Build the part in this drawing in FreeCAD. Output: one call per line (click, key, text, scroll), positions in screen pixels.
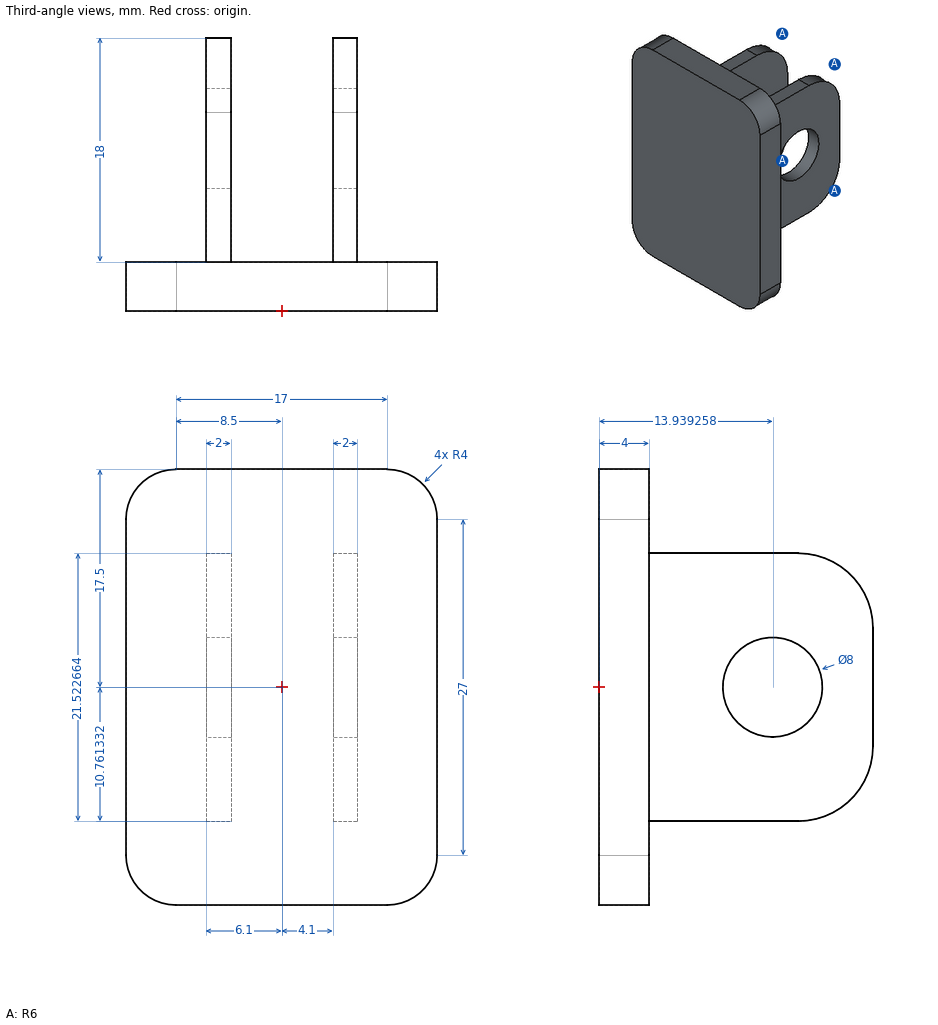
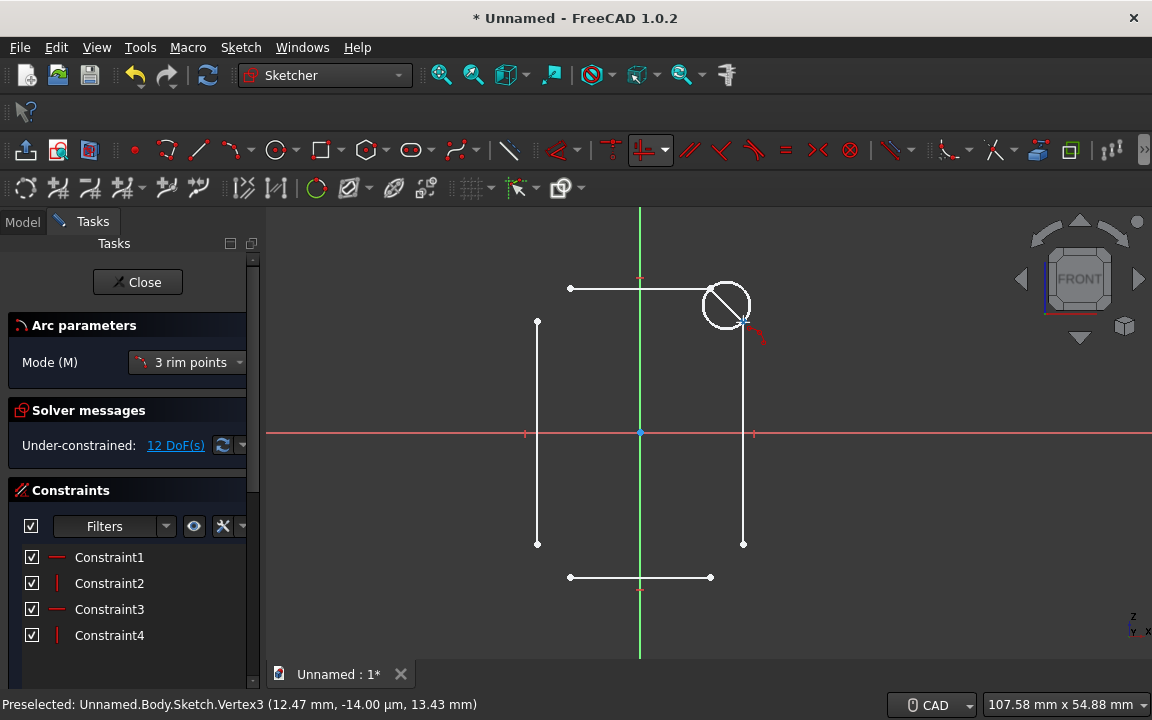
scroll(734, 298, up, 3)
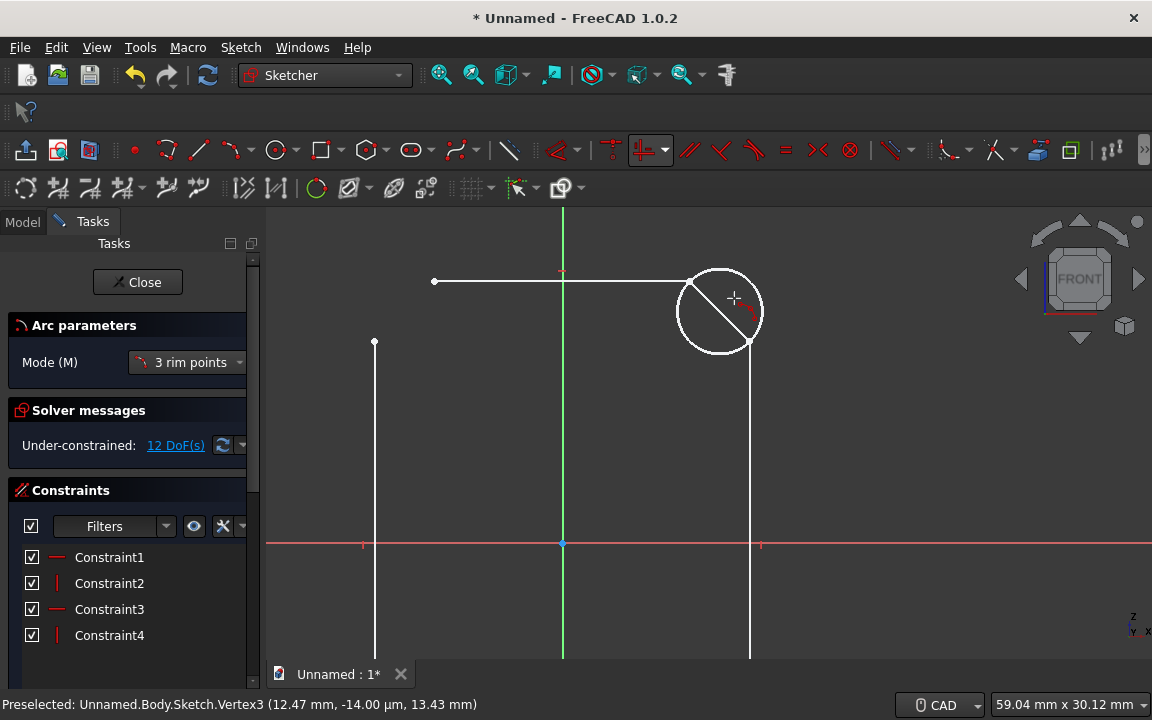
click(733, 298)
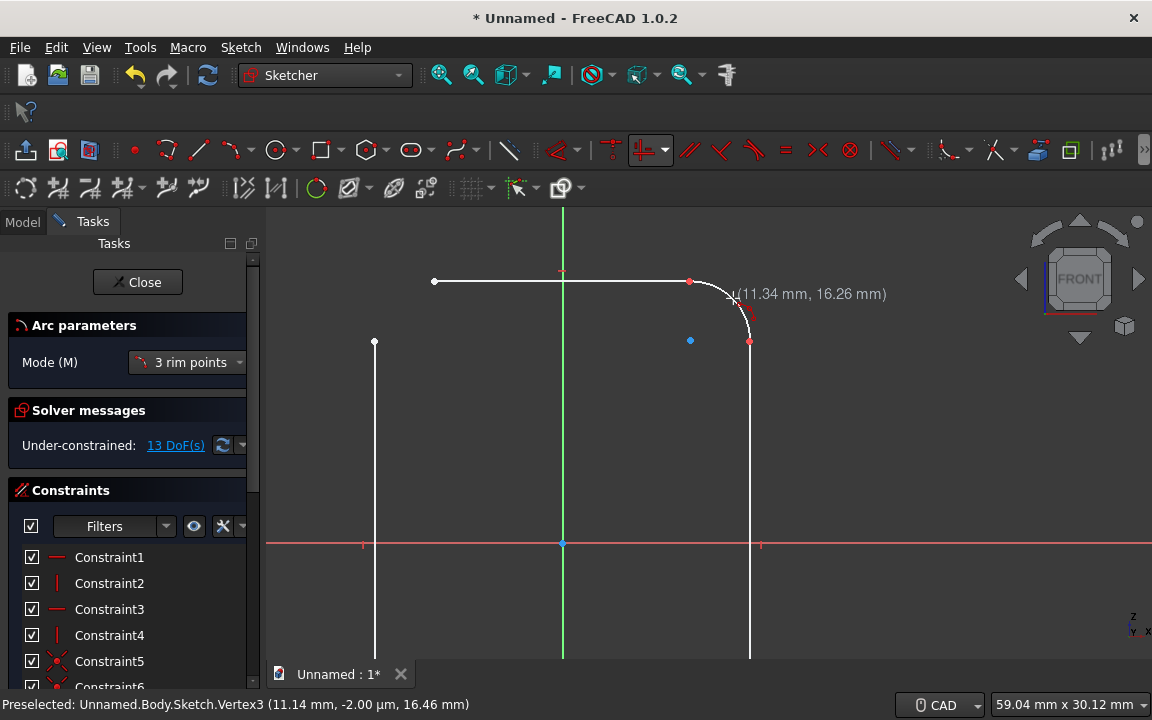
scroll(735, 299, down, 3)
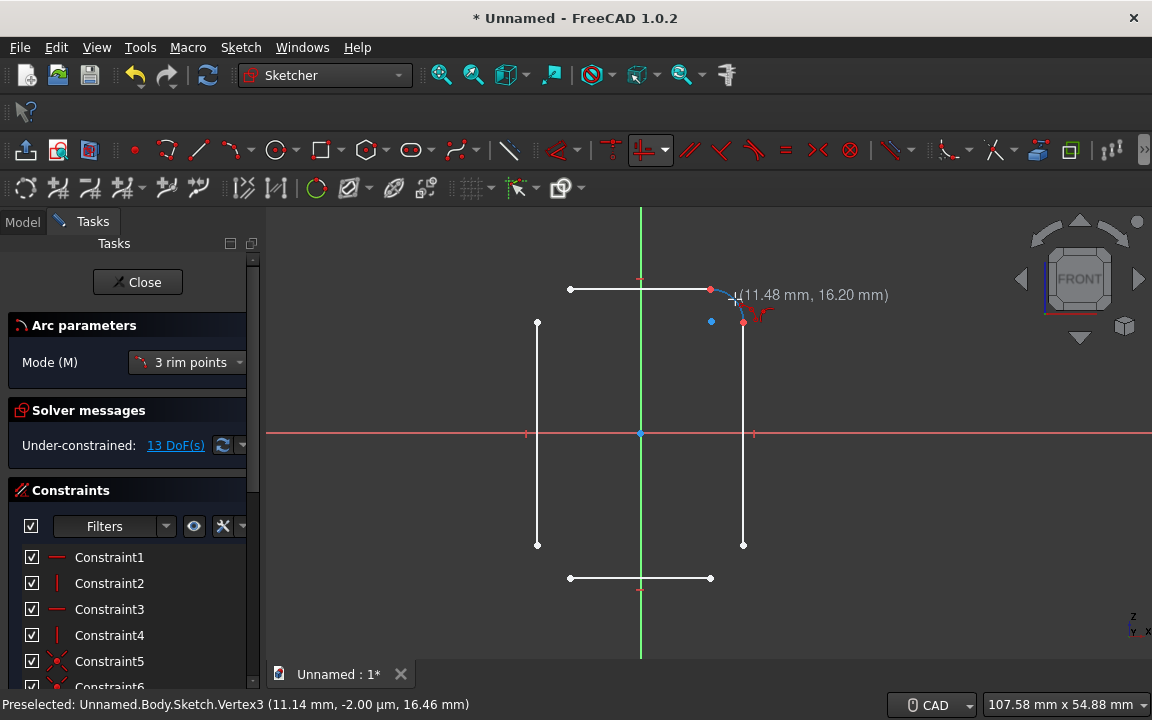
click(743, 545)
click(710, 578)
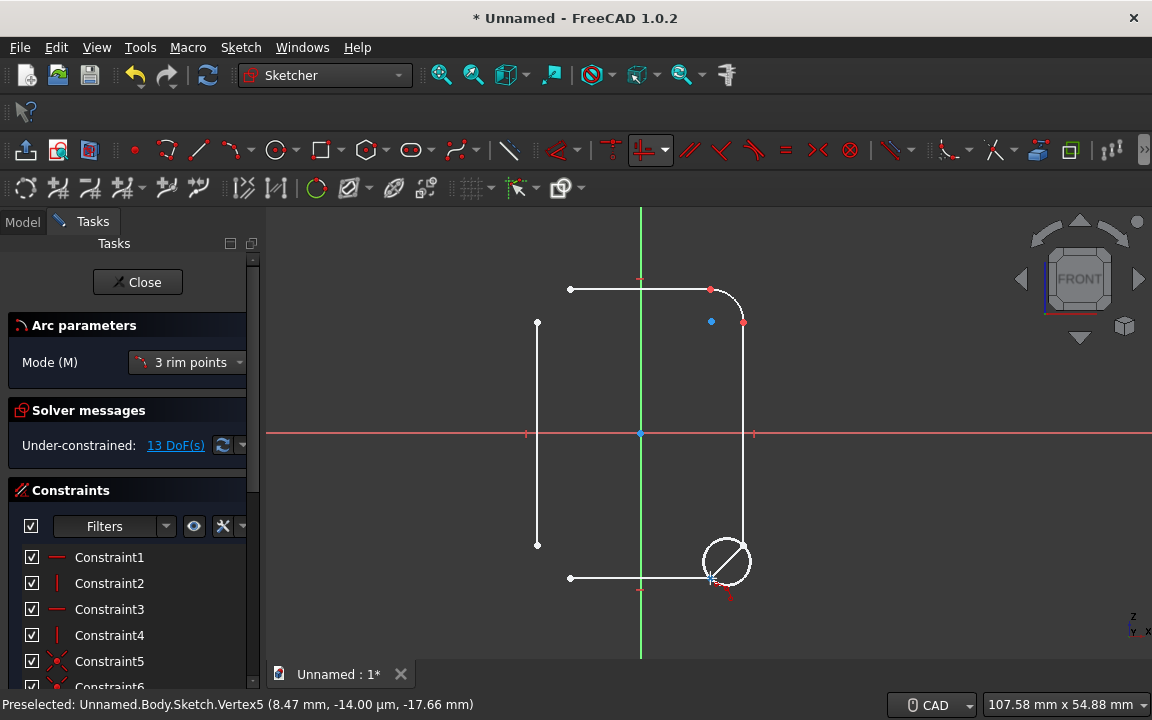
scroll(734, 568, up, 3)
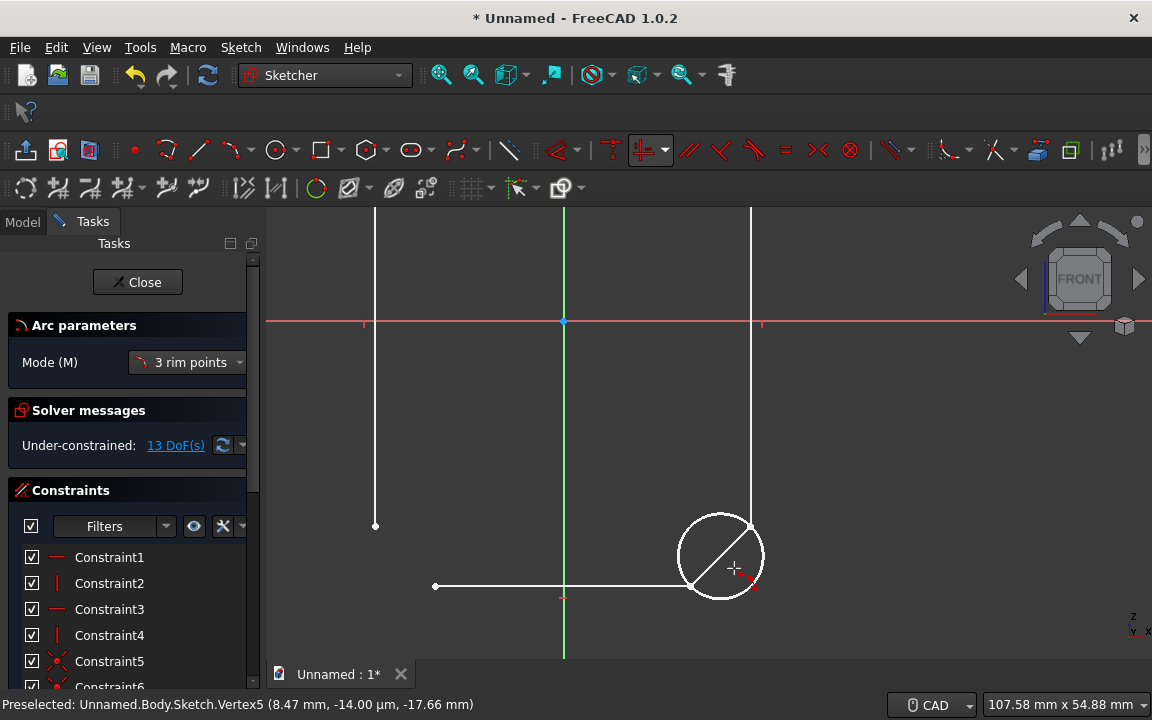
click(734, 566)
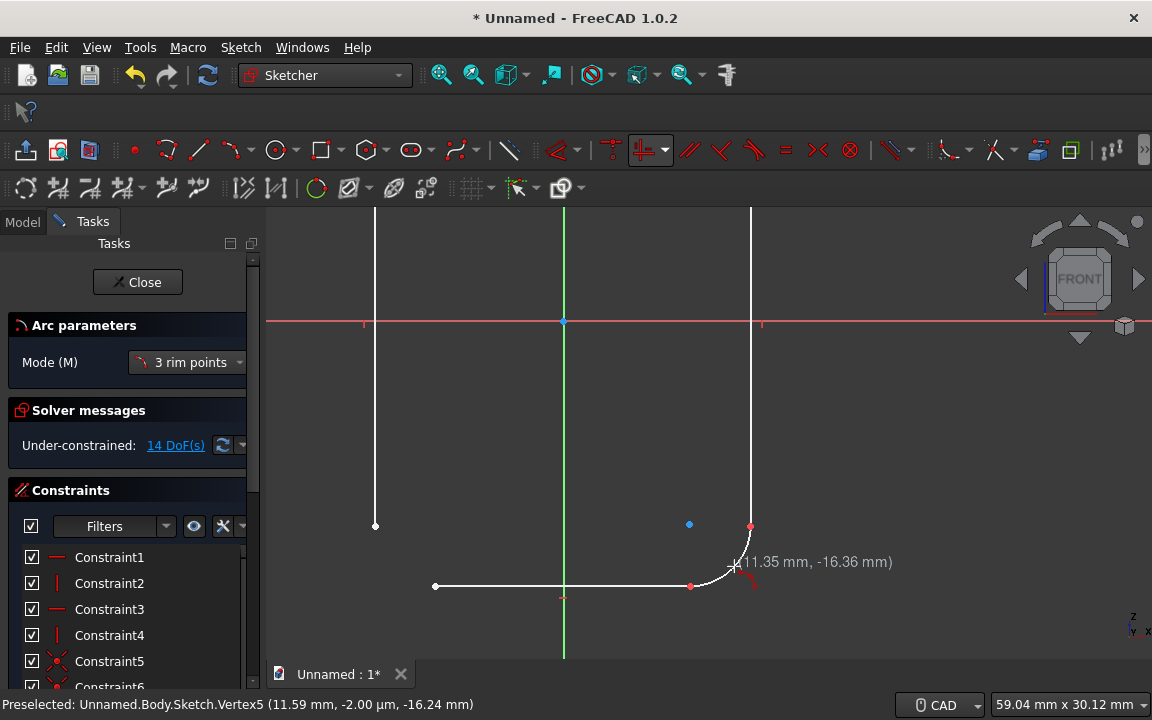
click(436, 586)
click(375, 526)
click(394, 566)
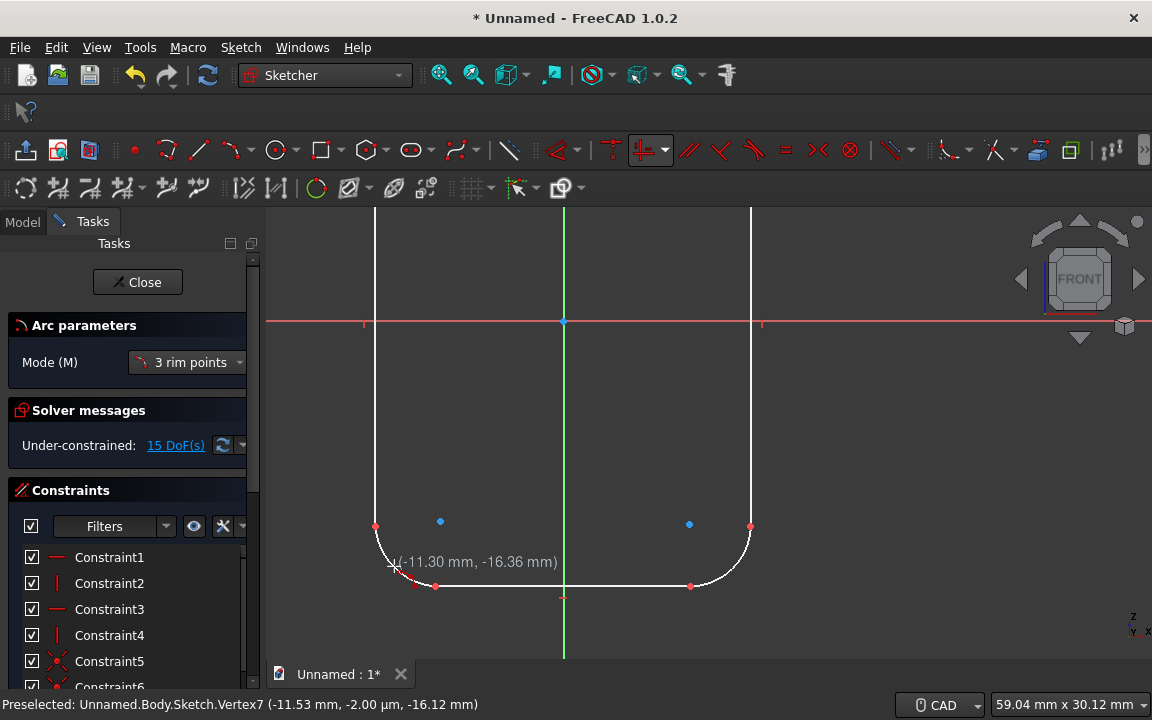
scroll(734, 569, down, 3)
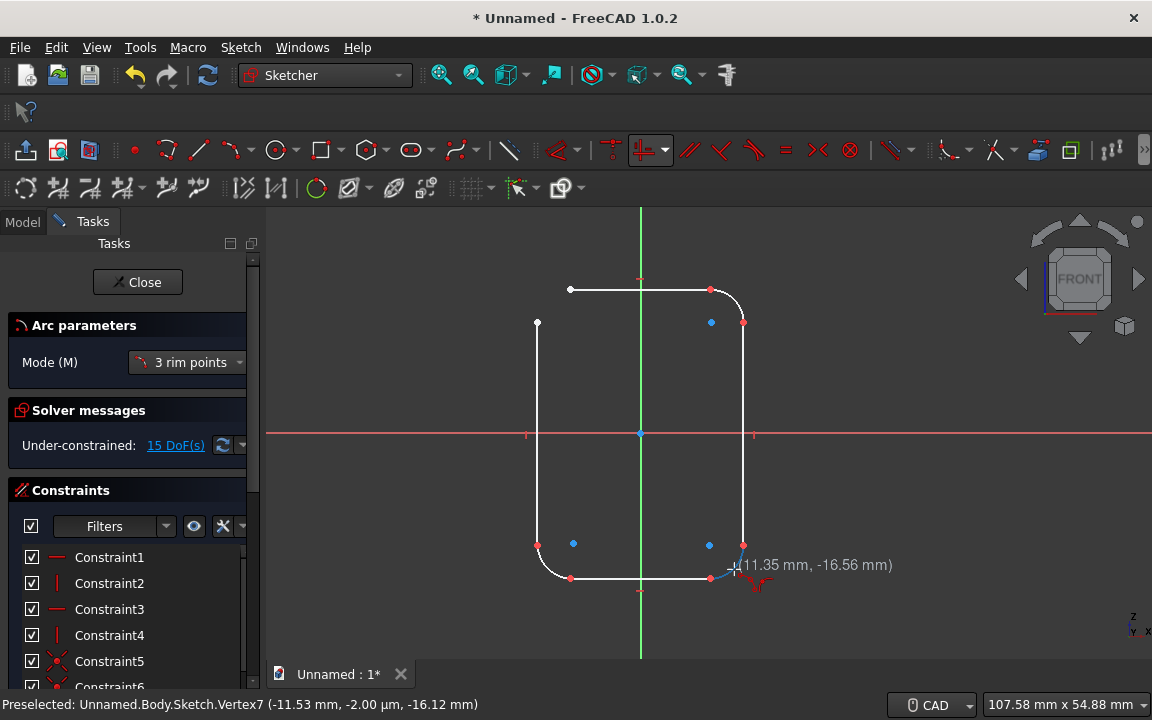
click(537, 323)
click(570, 290)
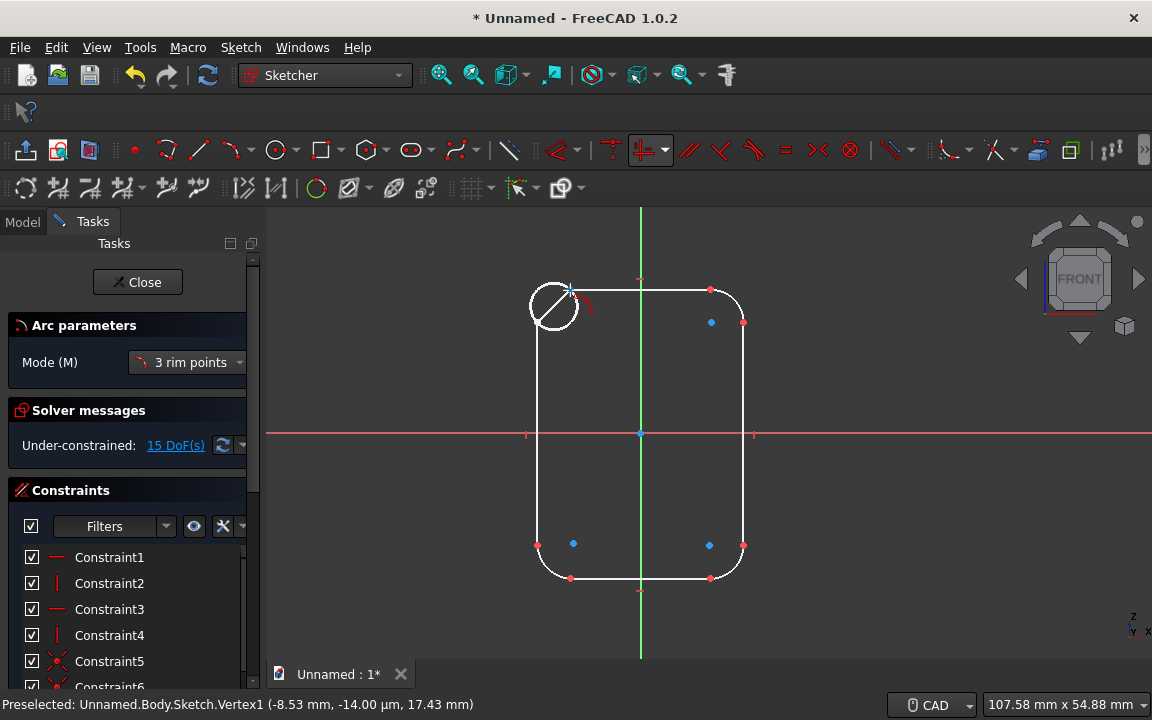
scroll(547, 299, up, 3)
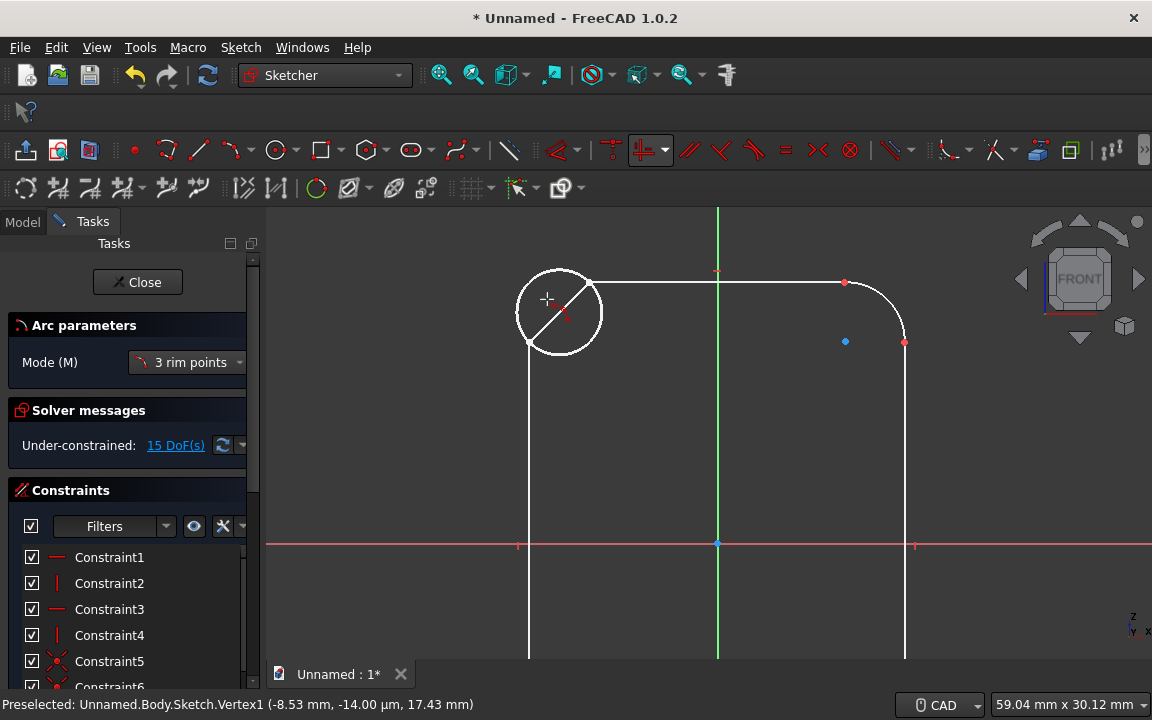
click(548, 299)
key(Escape)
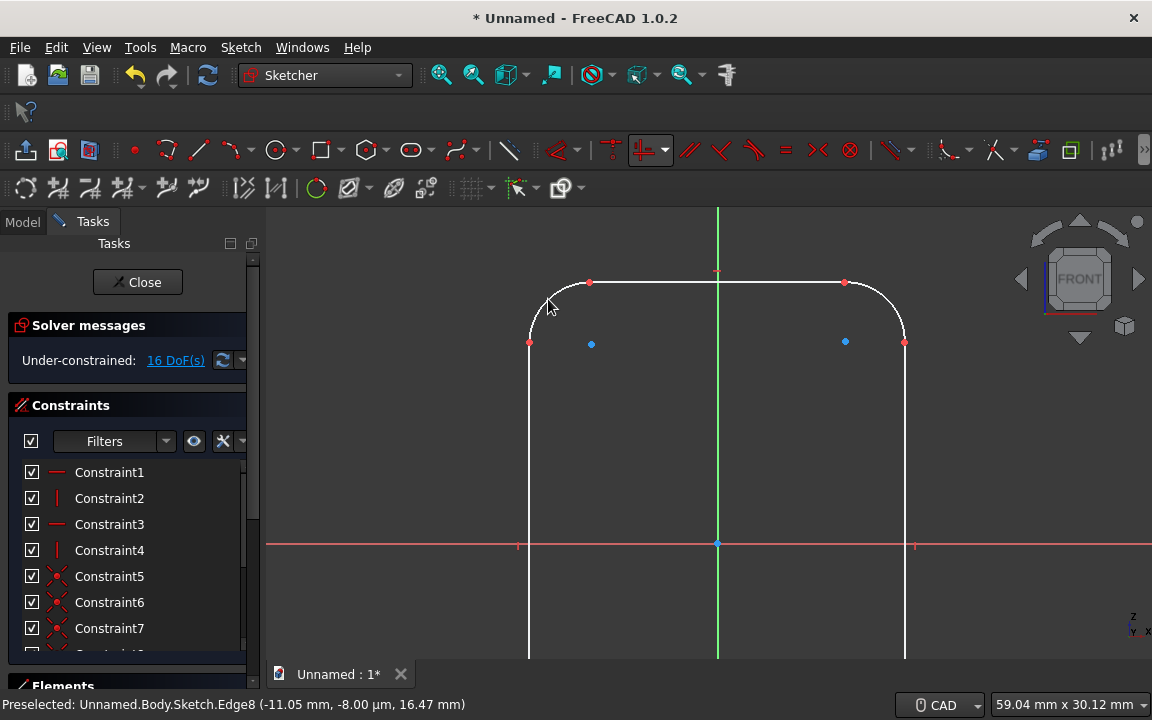
click(666, 282)